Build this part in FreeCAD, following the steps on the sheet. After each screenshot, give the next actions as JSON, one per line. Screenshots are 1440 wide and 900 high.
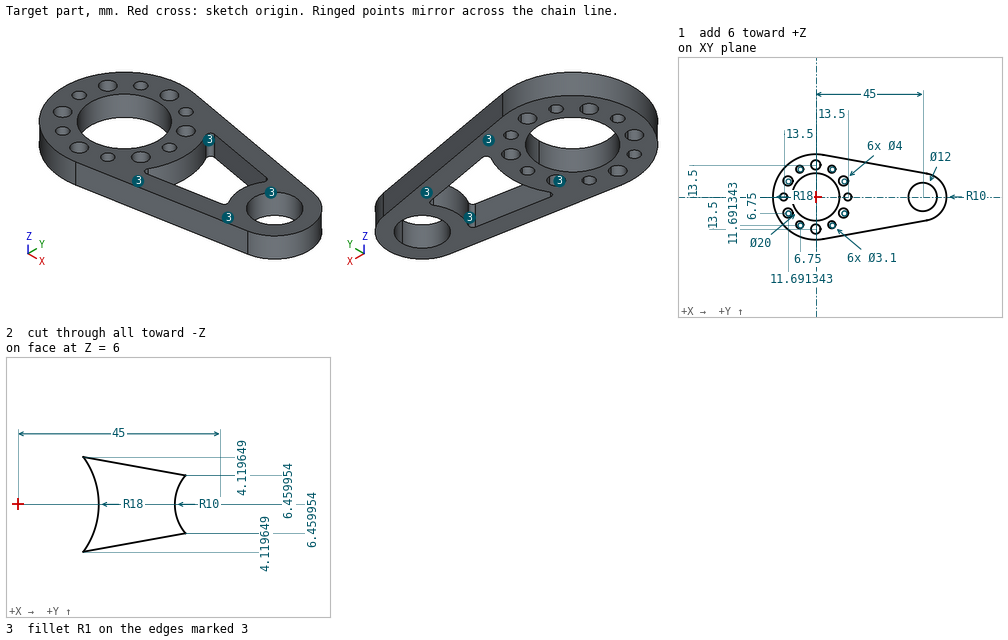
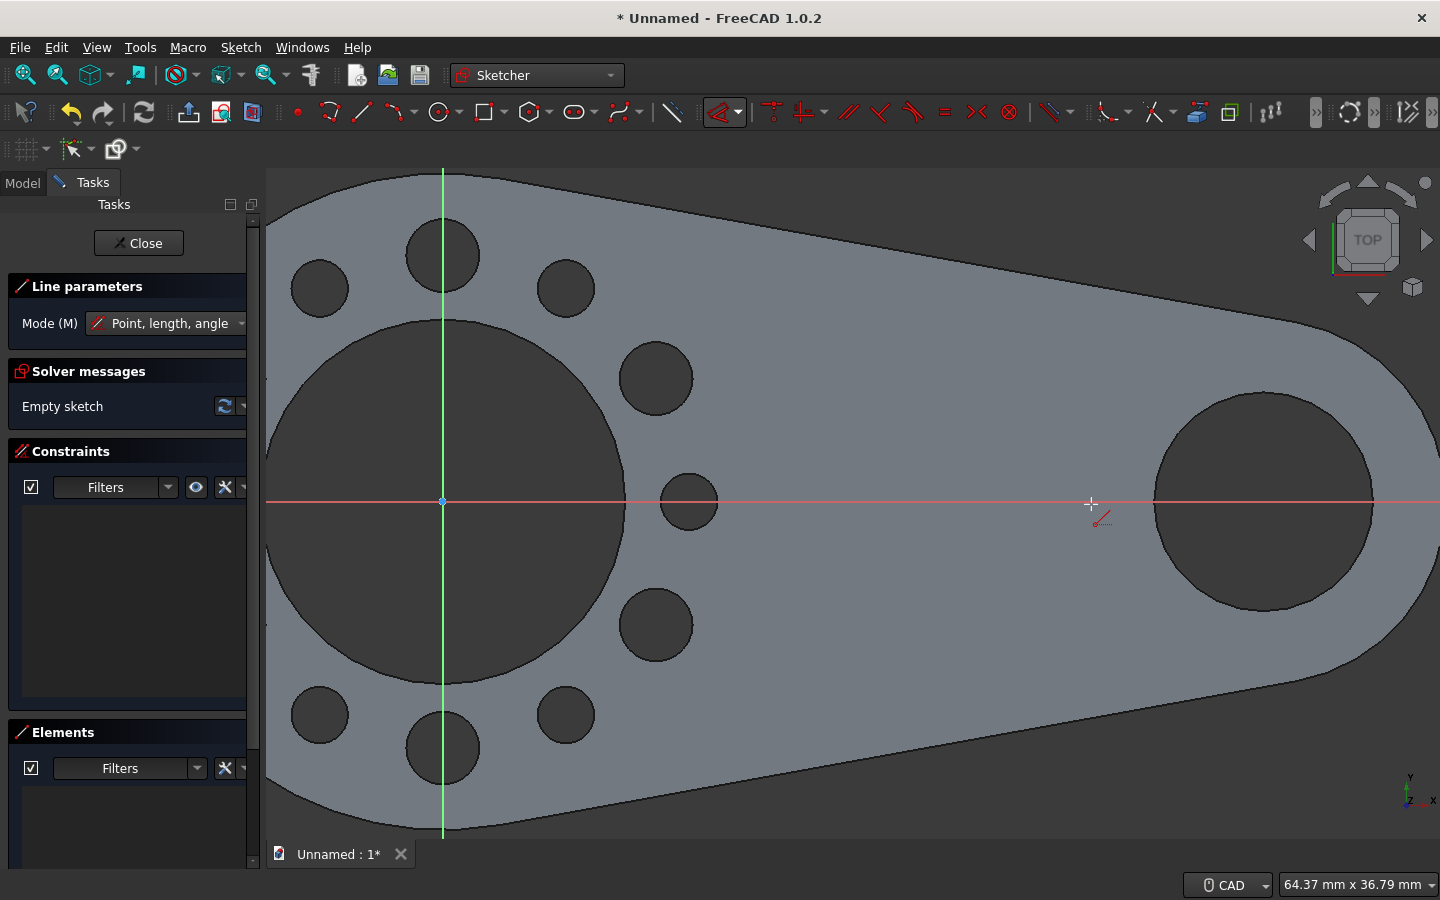
{"action": "left_click", "coordinate": [1124, 384]}
{"action": "left_click", "coordinate": [708, 309]}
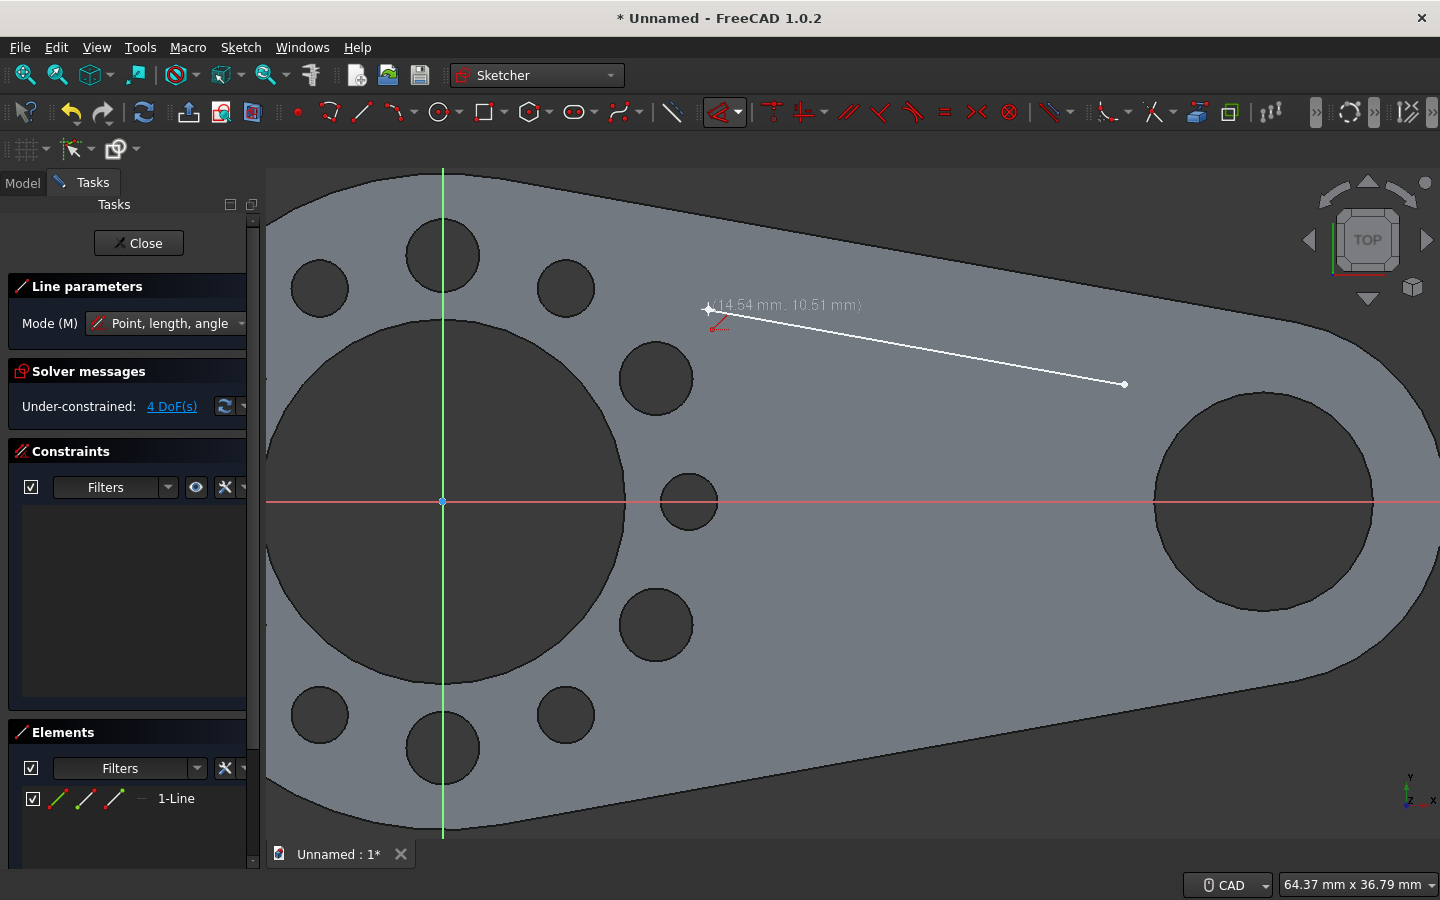
{"action": "left_click", "coordinate": [708, 695]}
{"action": "left_click", "coordinate": [1124, 620]}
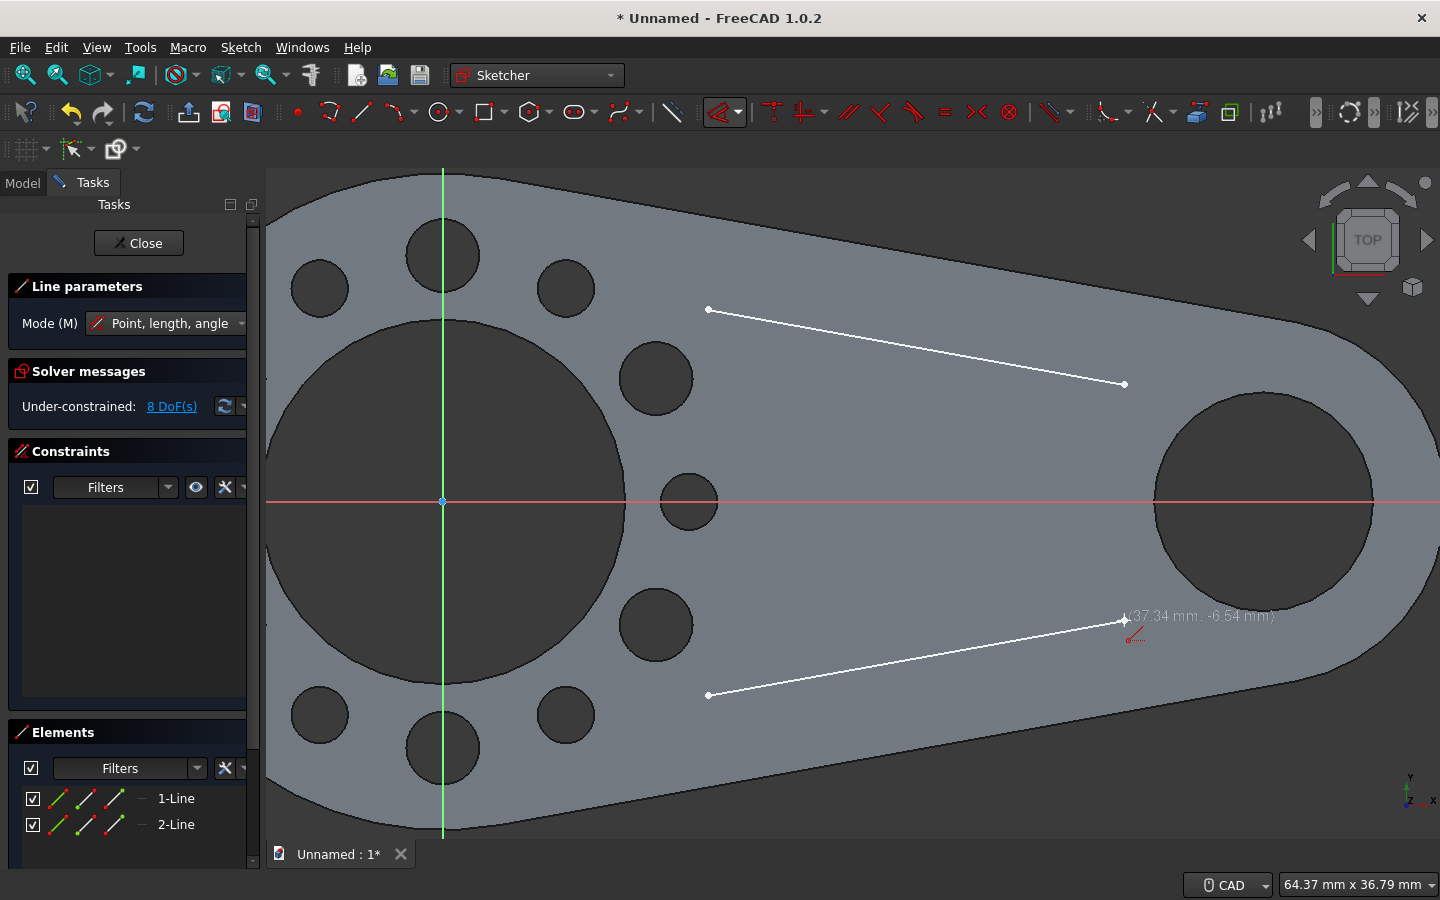
{"action": "left_click", "coordinate": [394, 112]}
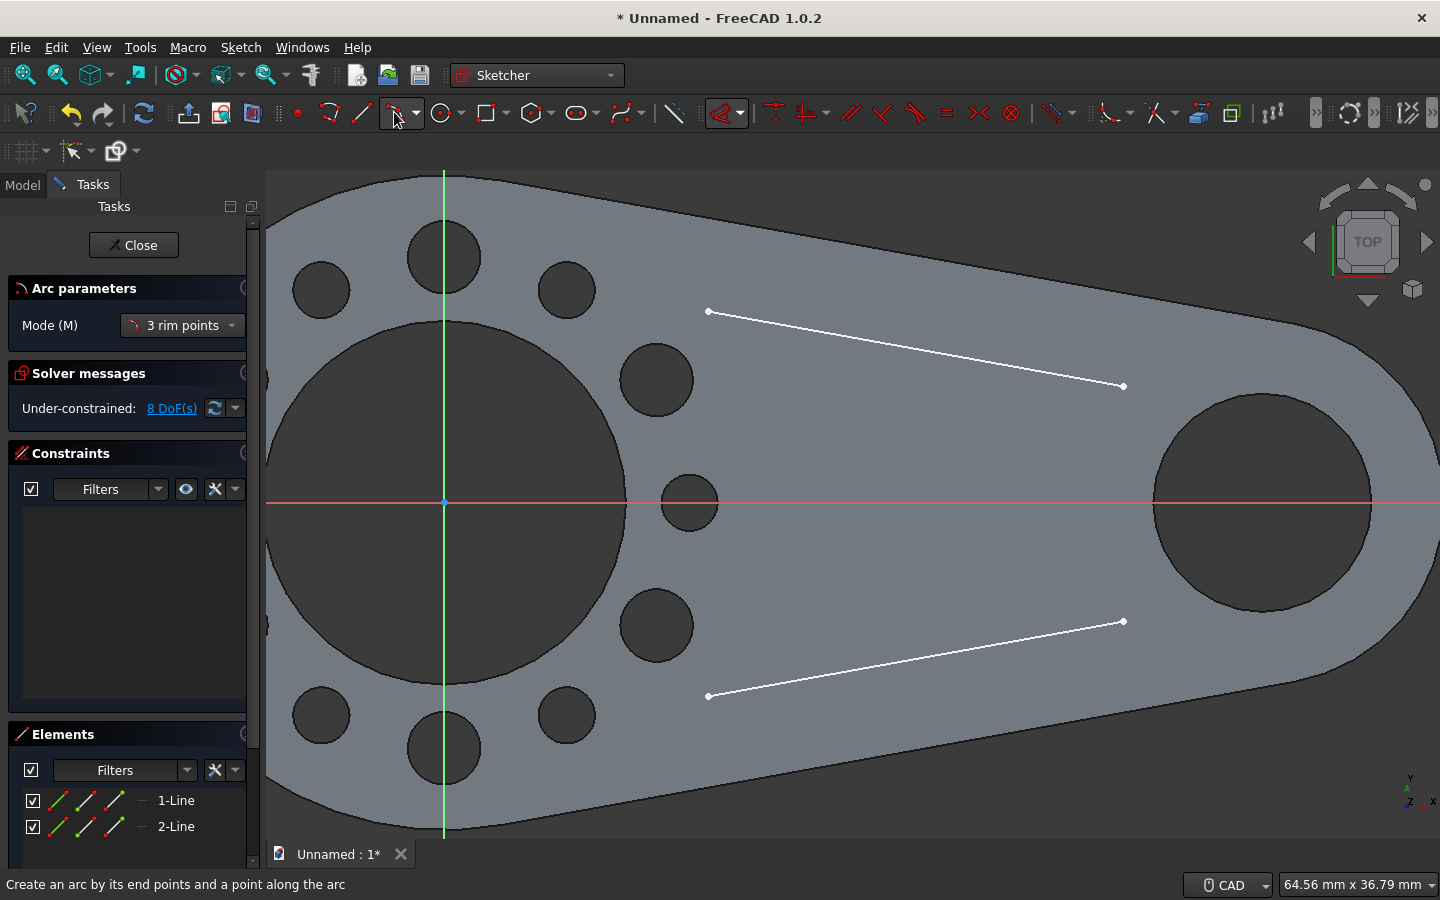
{"action": "left_click", "coordinate": [708, 312]}
{"action": "left_click", "coordinate": [708, 696]}
{"action": "left_click", "coordinate": [769, 544]}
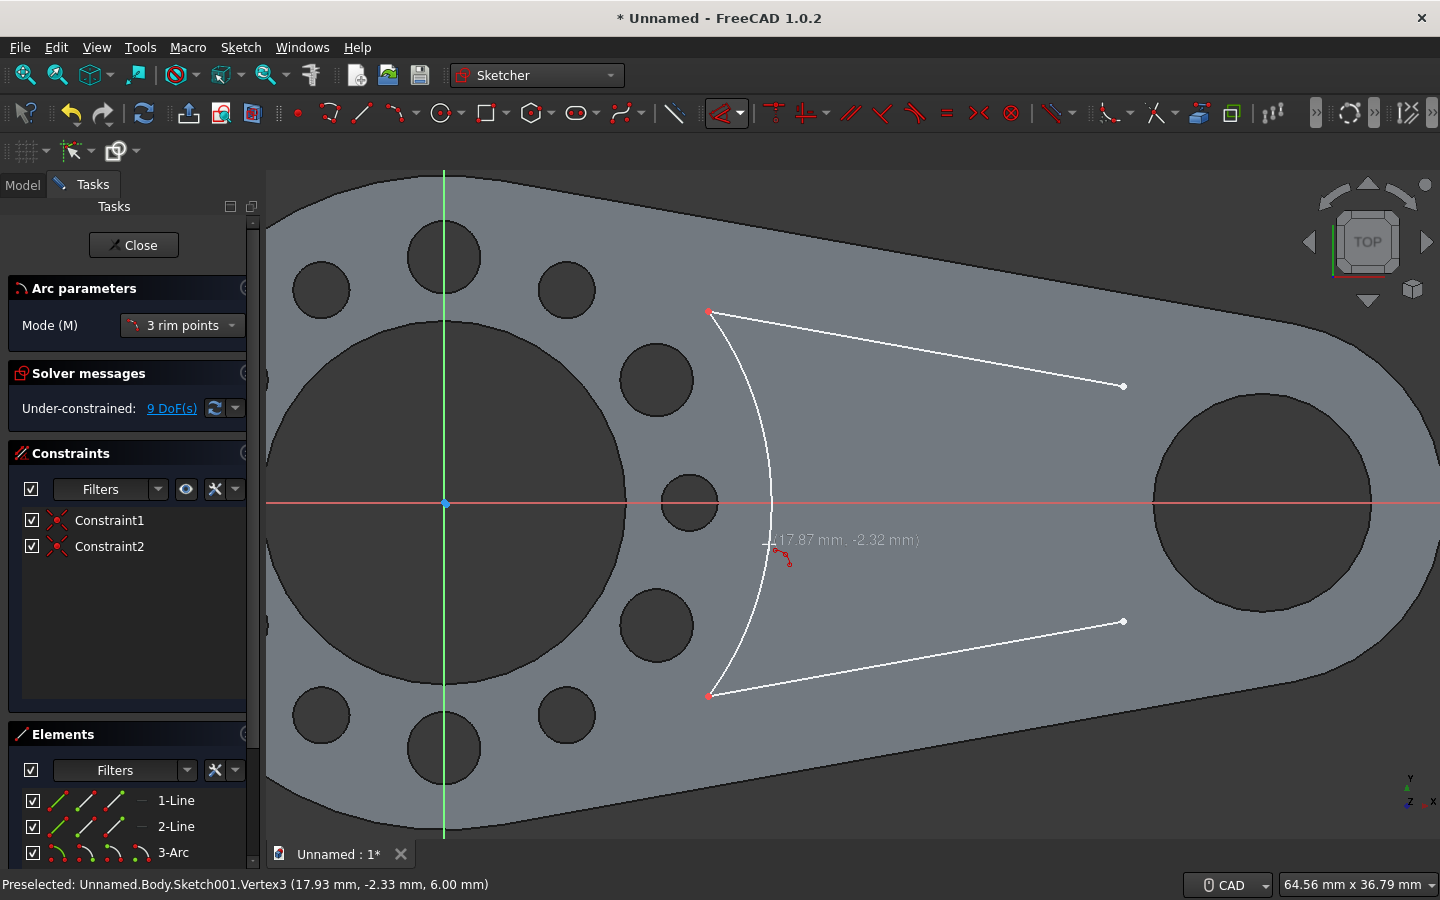
{"action": "left_click", "coordinate": [1123, 622]}
{"action": "left_click", "coordinate": [1123, 386]}
{"action": "left_click", "coordinate": [1082, 477]}
{"action": "key", "text": "Escape"}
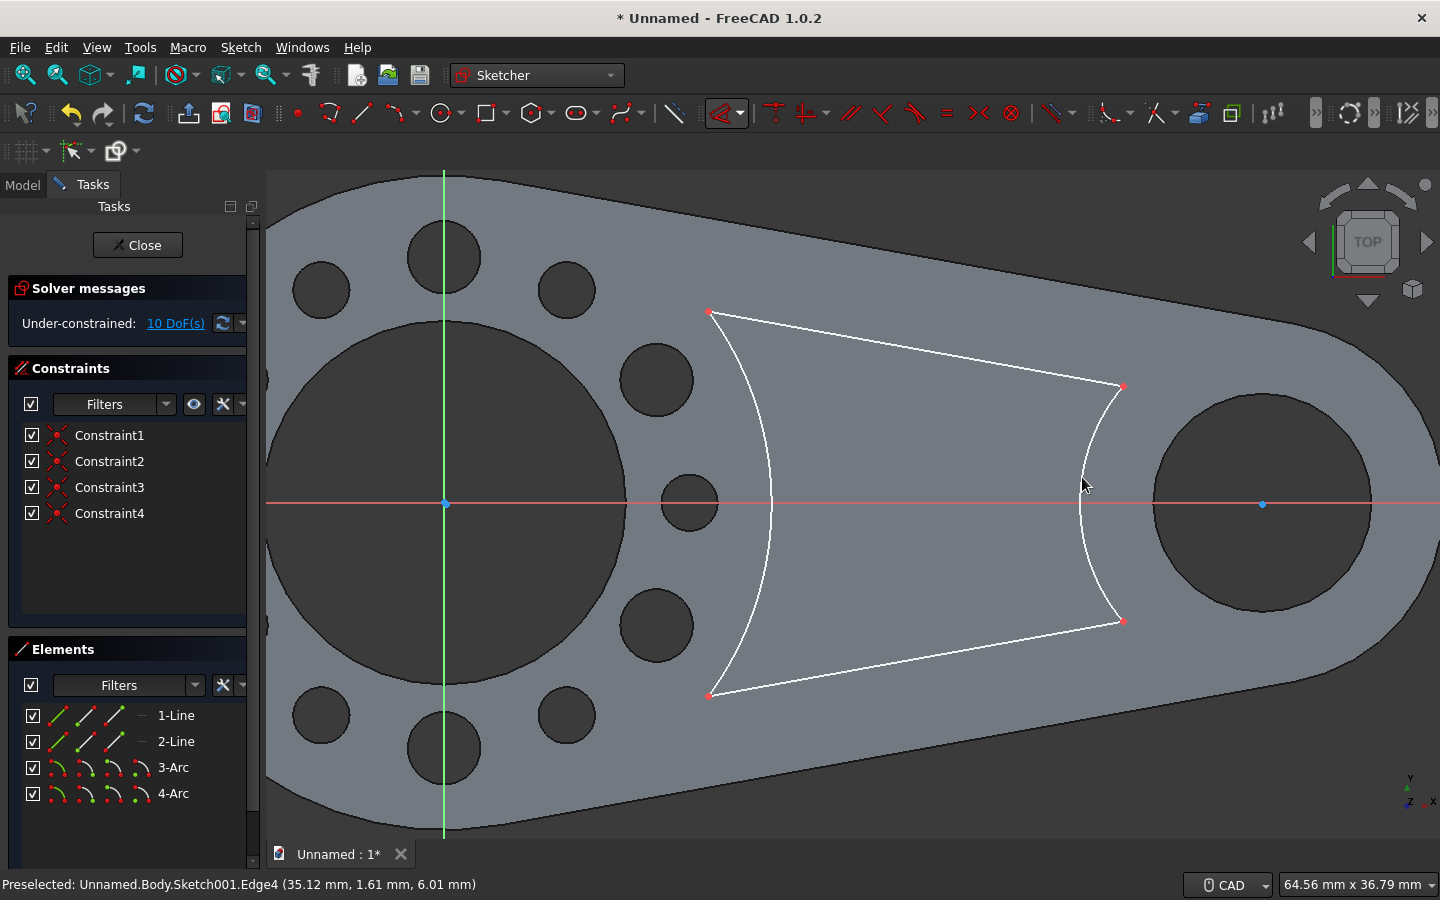
{"action": "left_click_drag", "start_coordinate": [434, 493], "coordinate": [457, 514]}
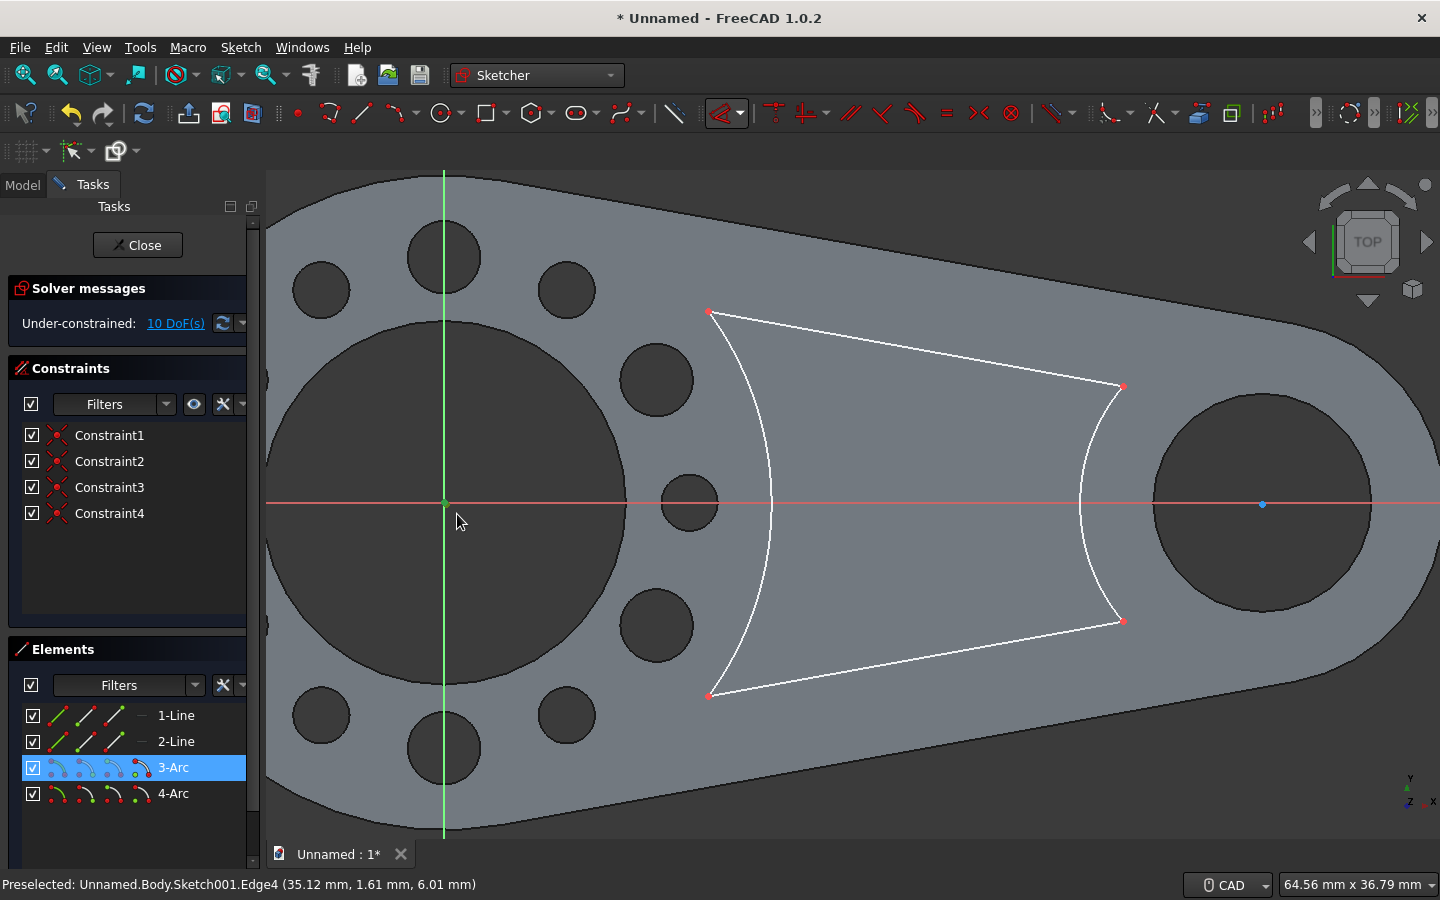
{"action": "left_click", "coordinate": [774, 114]}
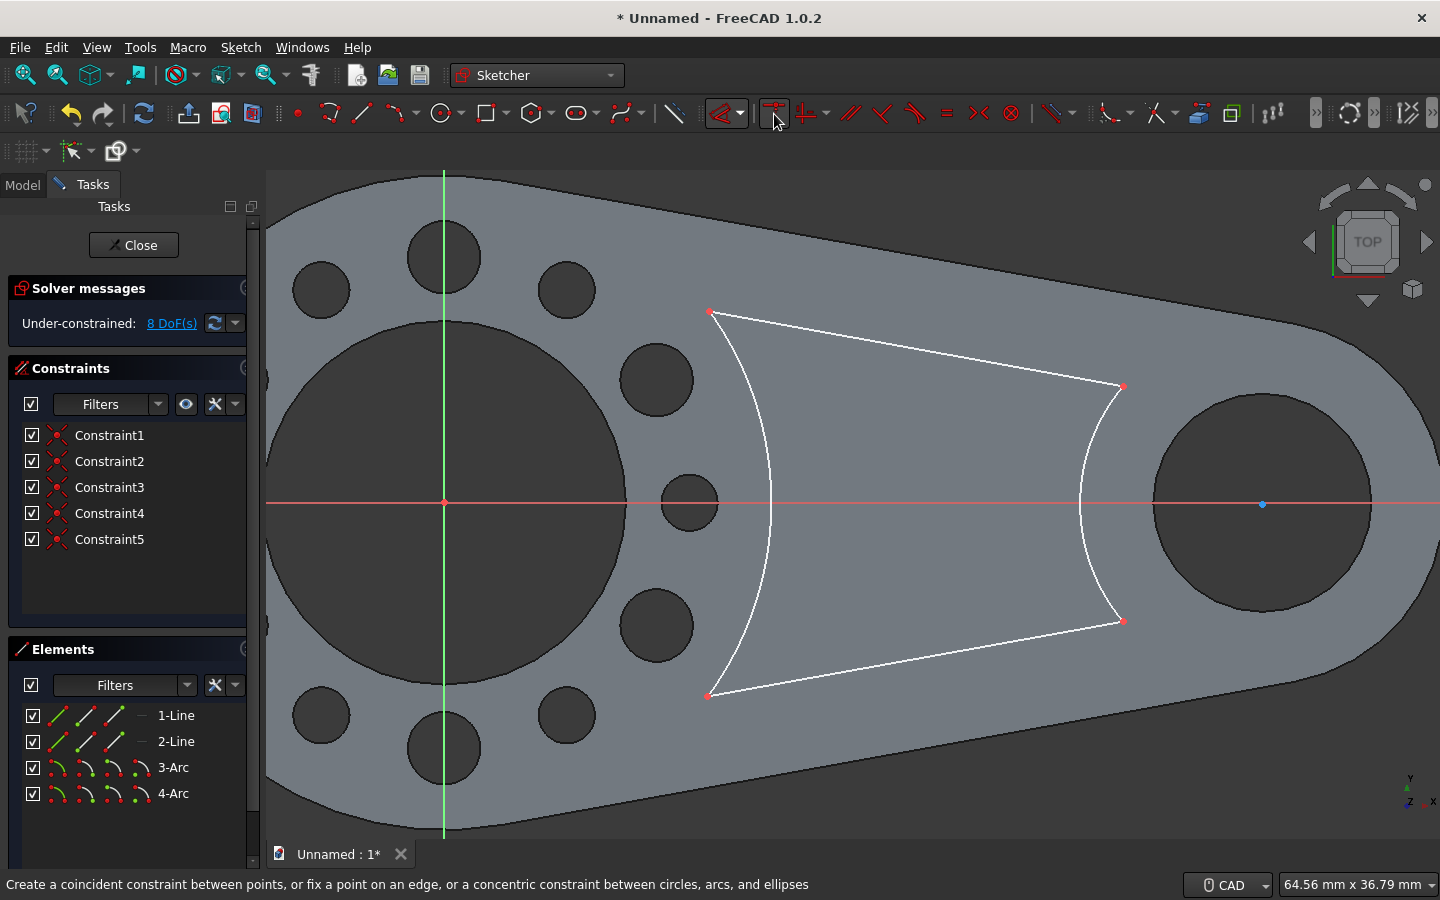
{"action": "left_click", "coordinate": [1262, 504]}